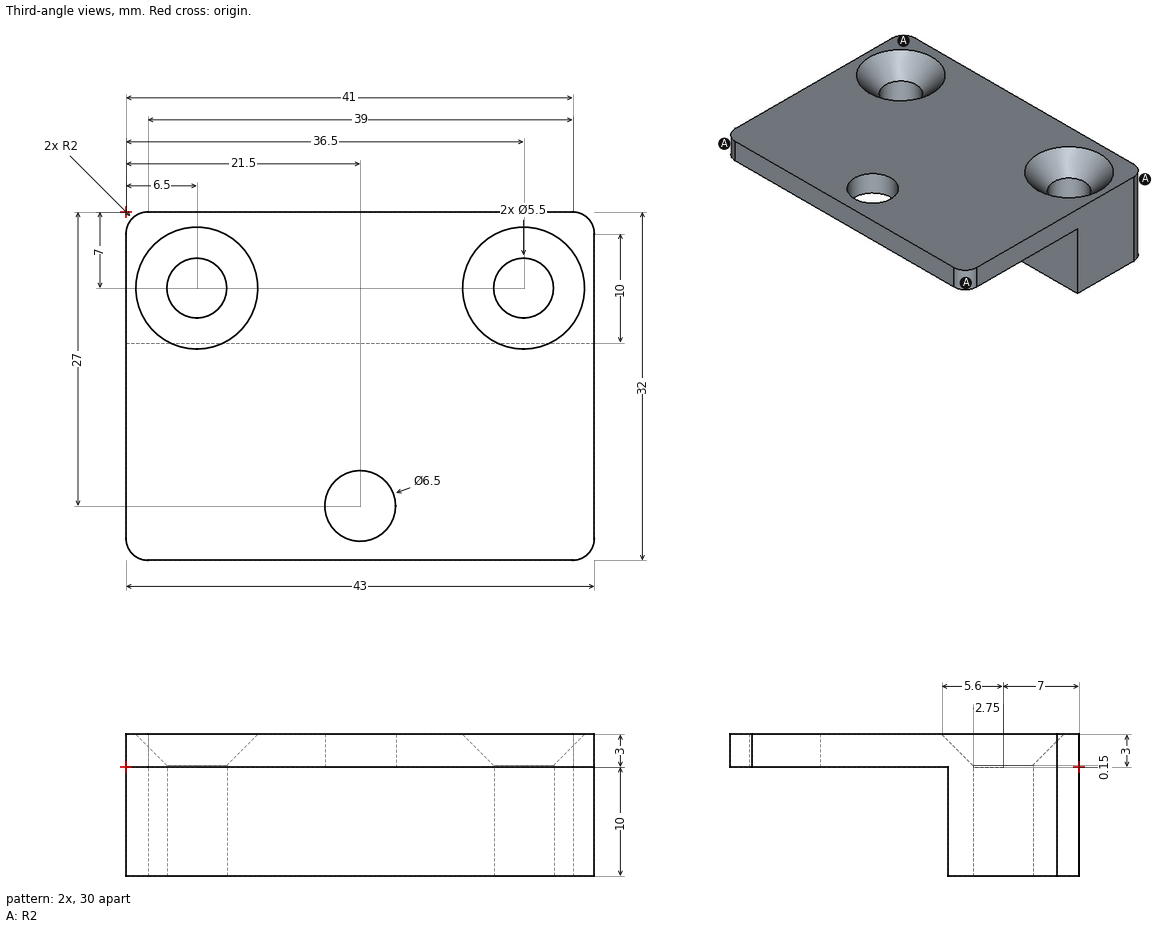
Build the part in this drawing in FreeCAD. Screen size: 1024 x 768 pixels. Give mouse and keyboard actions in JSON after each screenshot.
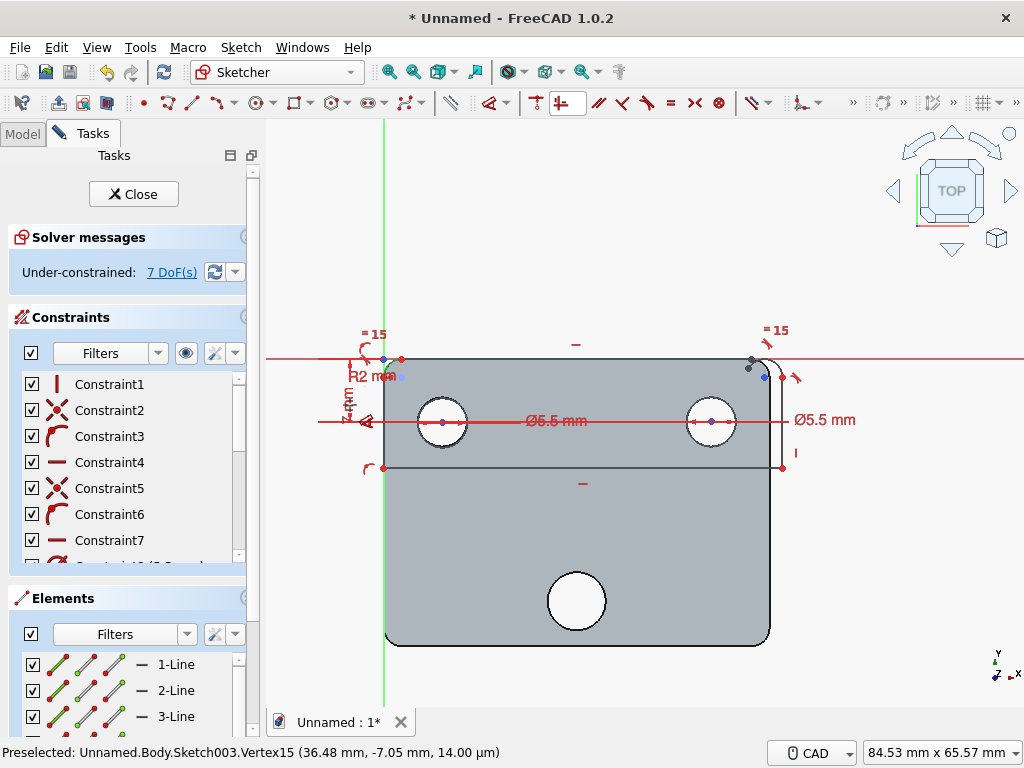
{"action": "left_click", "coordinate": [443, 423]}
{"action": "left_click", "coordinate": [477, 391]}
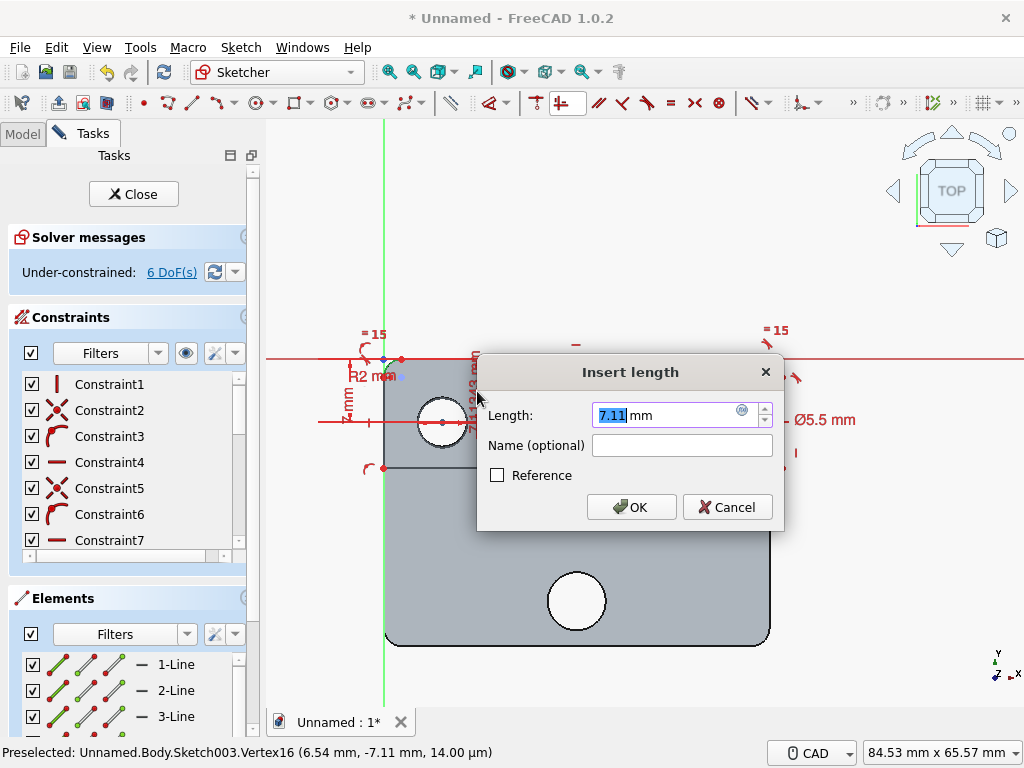
{"action": "type", "text": "7"}
{"action": "key", "text": "Return"}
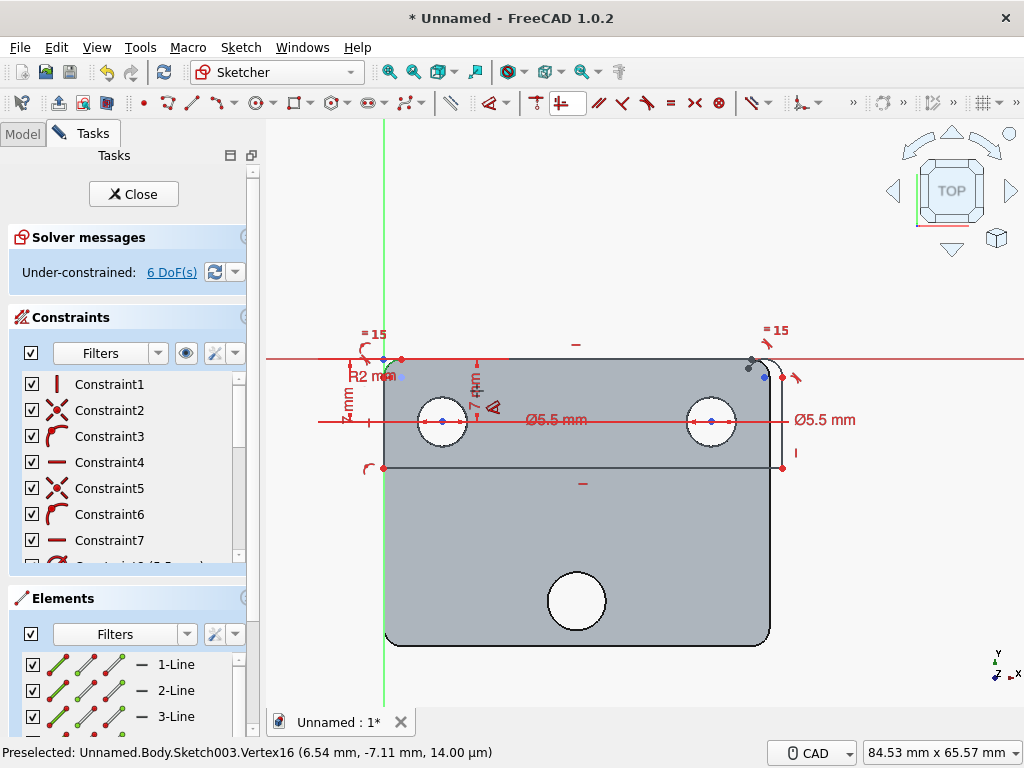
{"action": "left_click", "coordinate": [782, 405]}
{"action": "left_click", "coordinate": [816, 423]}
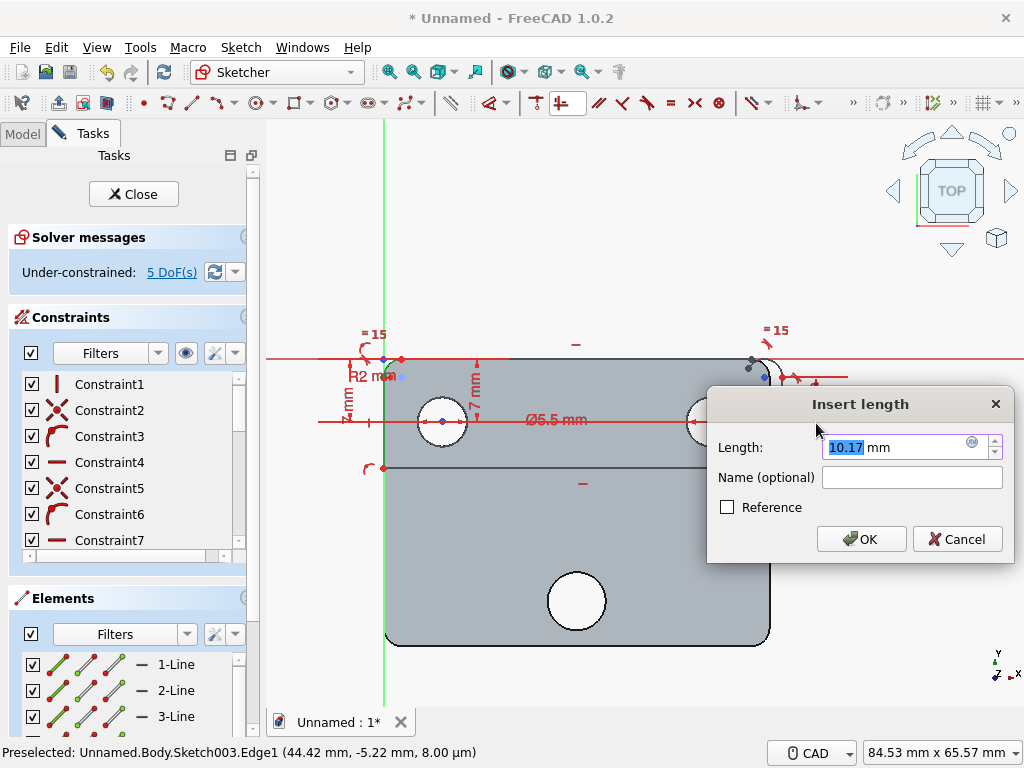
{"action": "type", "text": "10"}
{"action": "key", "text": "Return"}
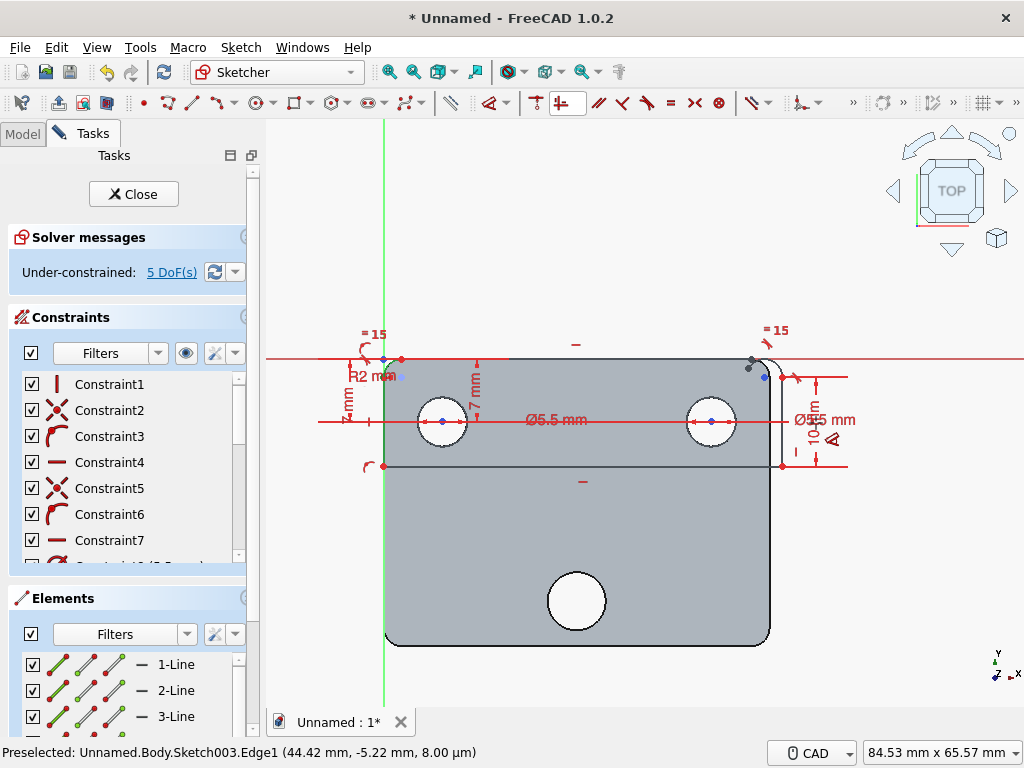
{"action": "left_click", "coordinate": [663, 467]}
{"action": "left_click", "coordinate": [583, 501]}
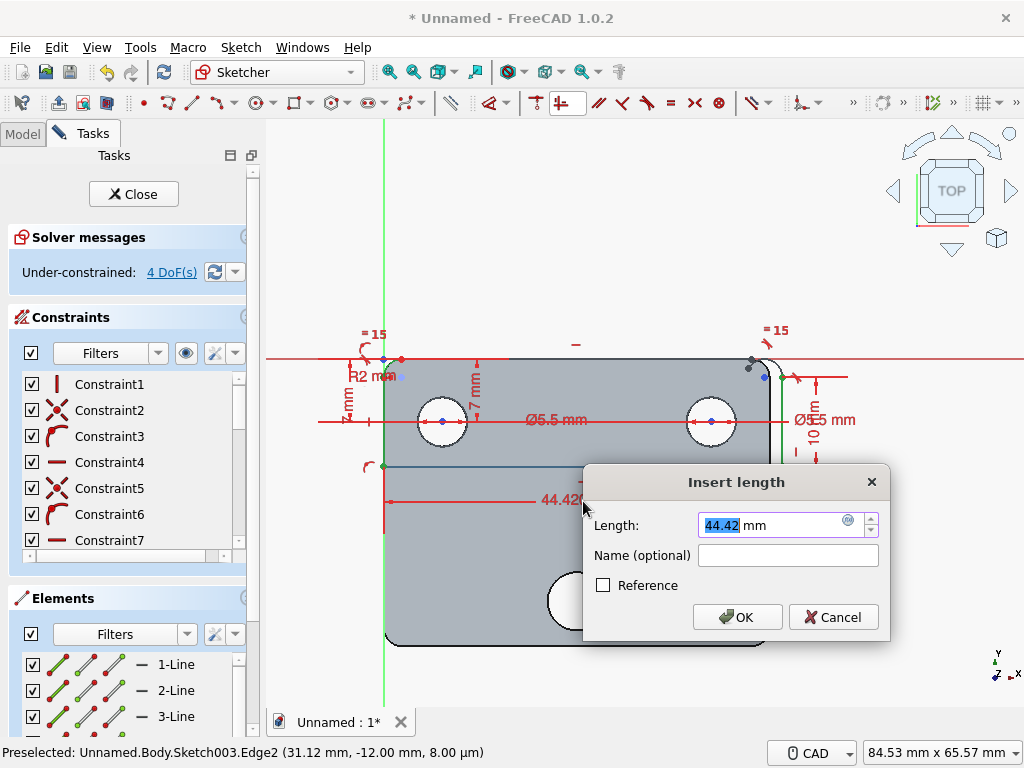
{"action": "type", "text": "43"}
{"action": "key", "text": "Return"}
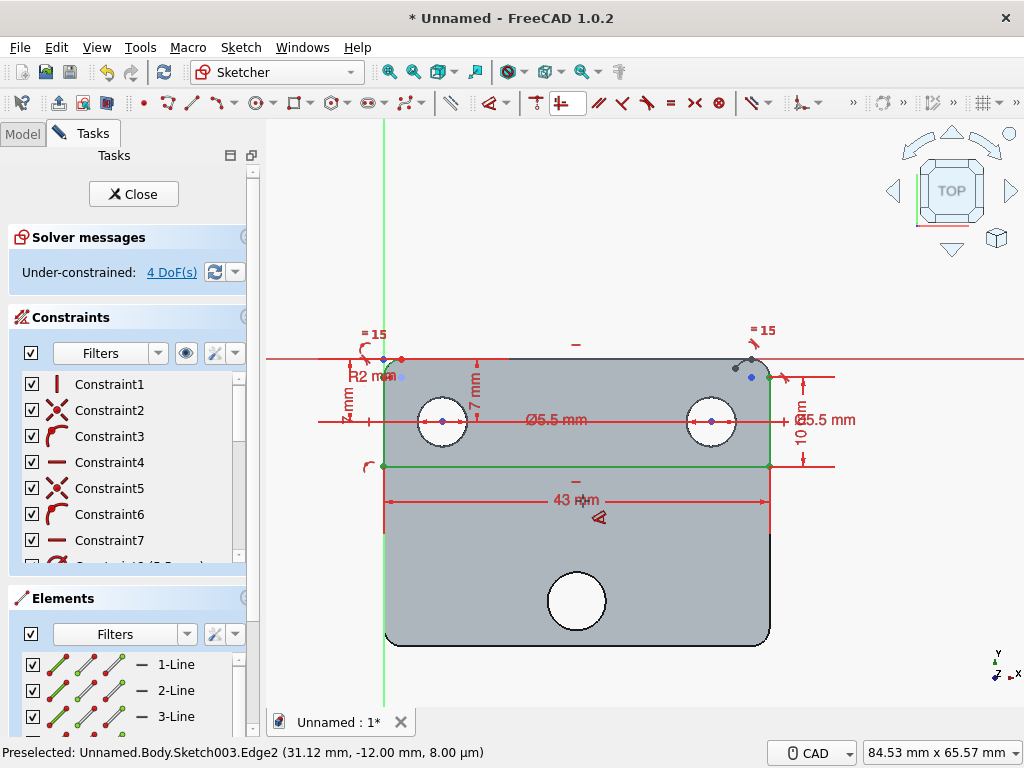
{"action": "left_click", "coordinate": [507, 359]}
{"action": "left_click", "coordinate": [577, 325]}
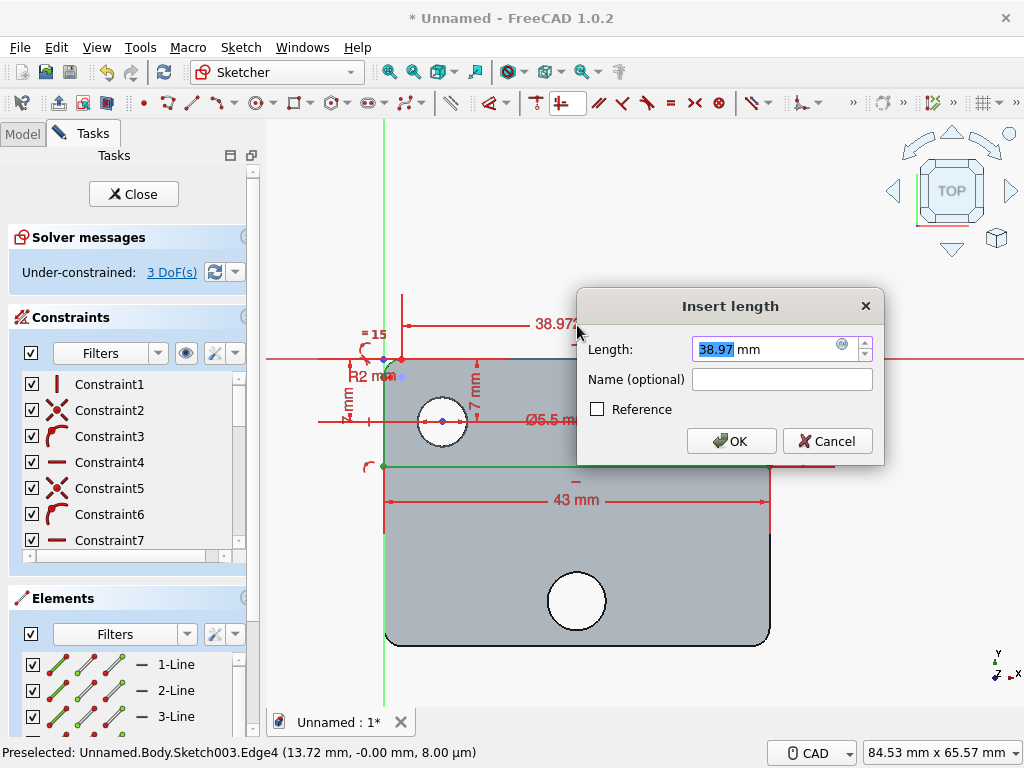
{"action": "type", "text": "39"}
{"action": "key", "text": "Return"}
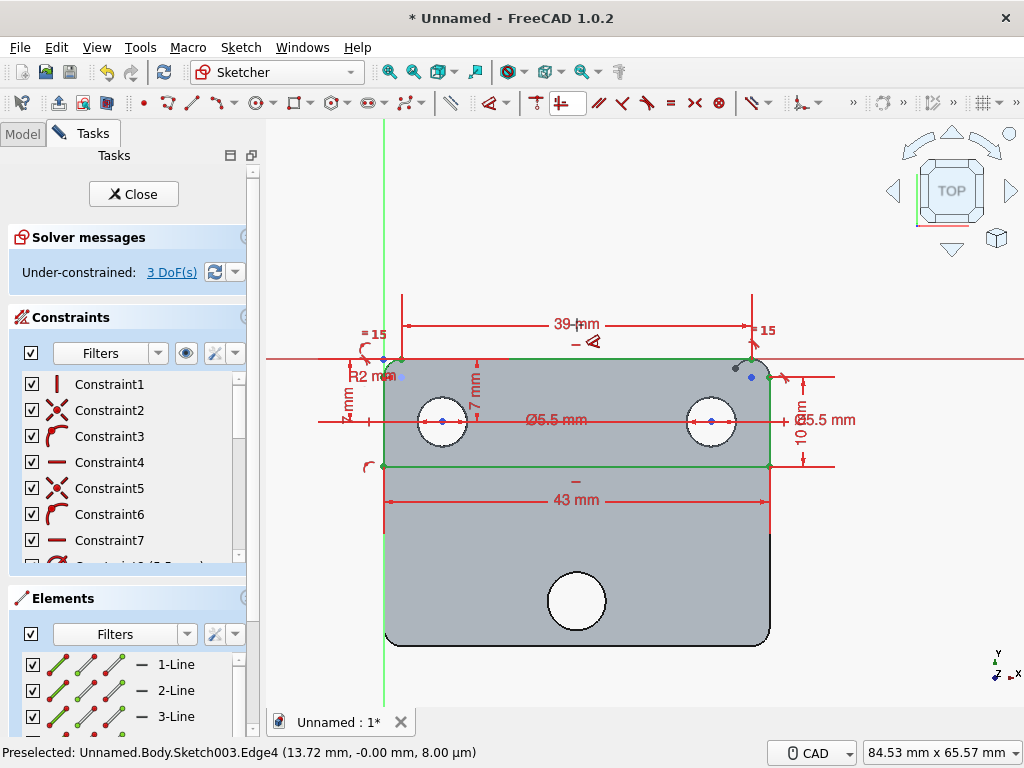
{"action": "left_click", "coordinate": [736, 369]}
{"action": "left_click", "coordinate": [479, 325]}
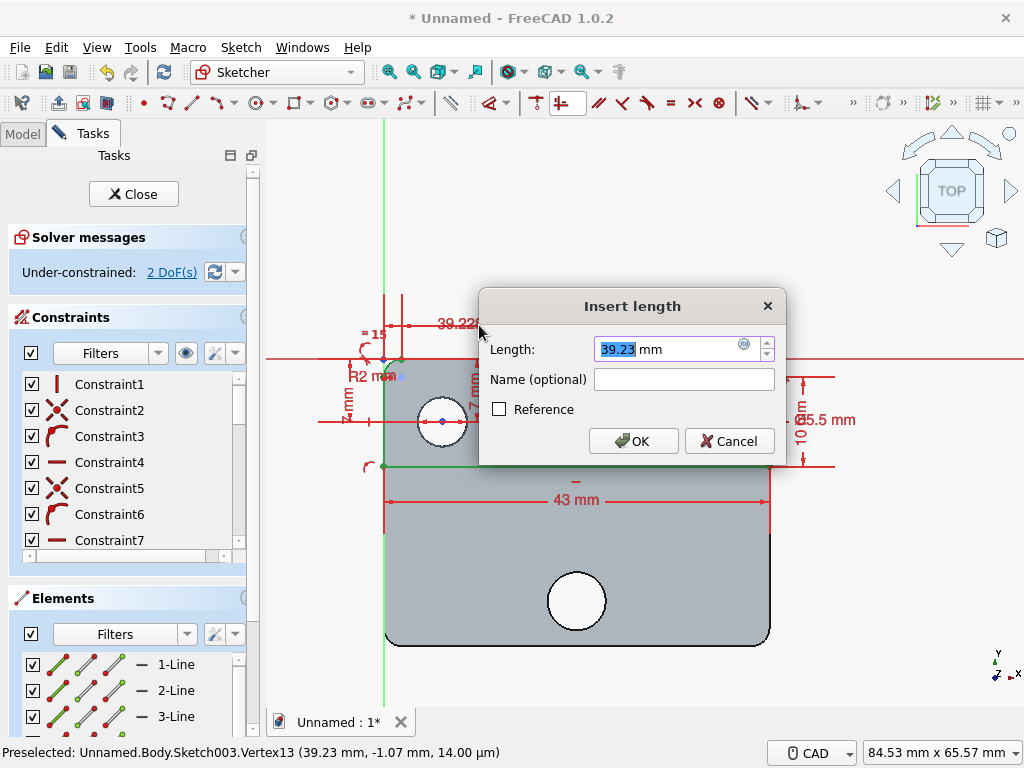
{"action": "type", "text": "41"}
{"action": "key", "text": "Return"}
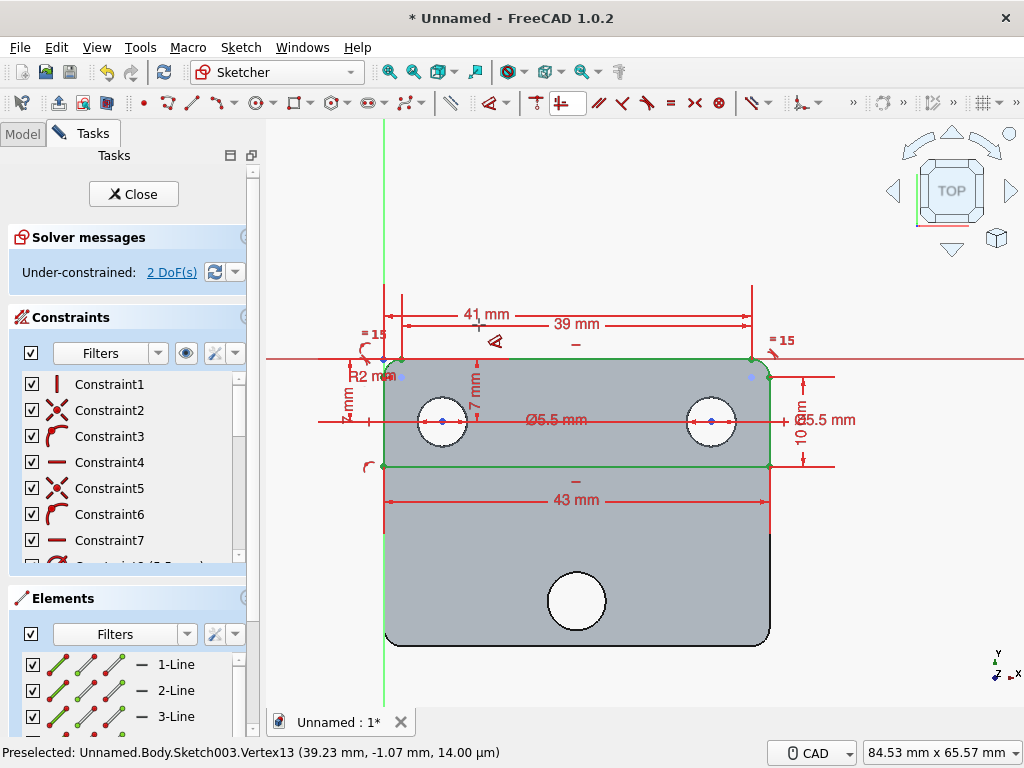
{"action": "left_click", "coordinate": [443, 422]}
{"action": "left_click", "coordinate": [400, 325]}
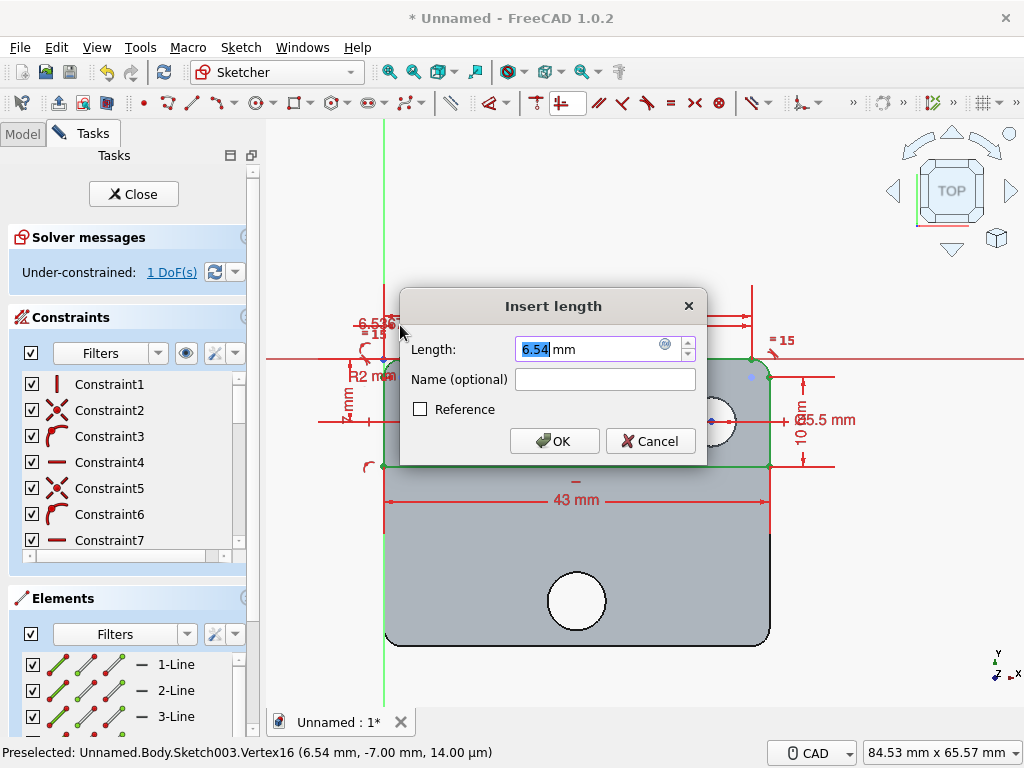
{"action": "type", "text": "6.5"}
{"action": "key", "text": "Return"}